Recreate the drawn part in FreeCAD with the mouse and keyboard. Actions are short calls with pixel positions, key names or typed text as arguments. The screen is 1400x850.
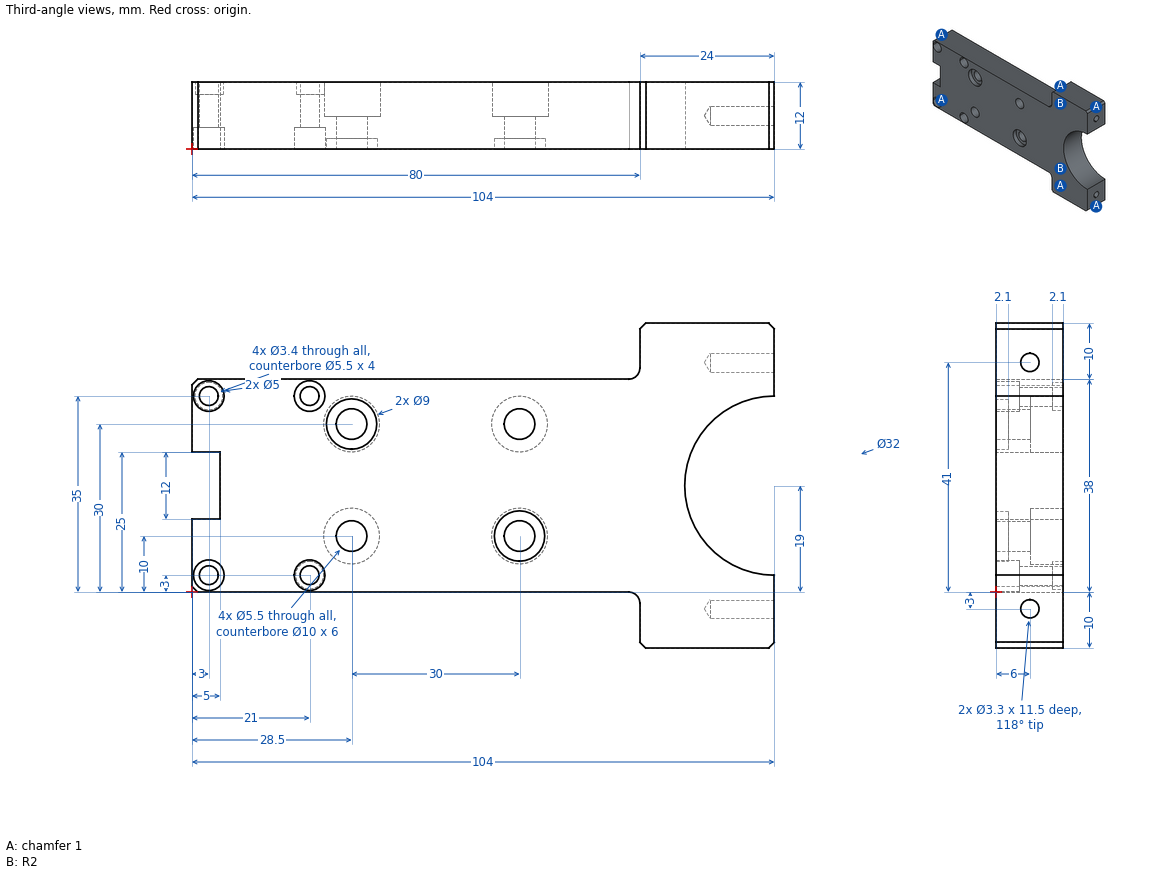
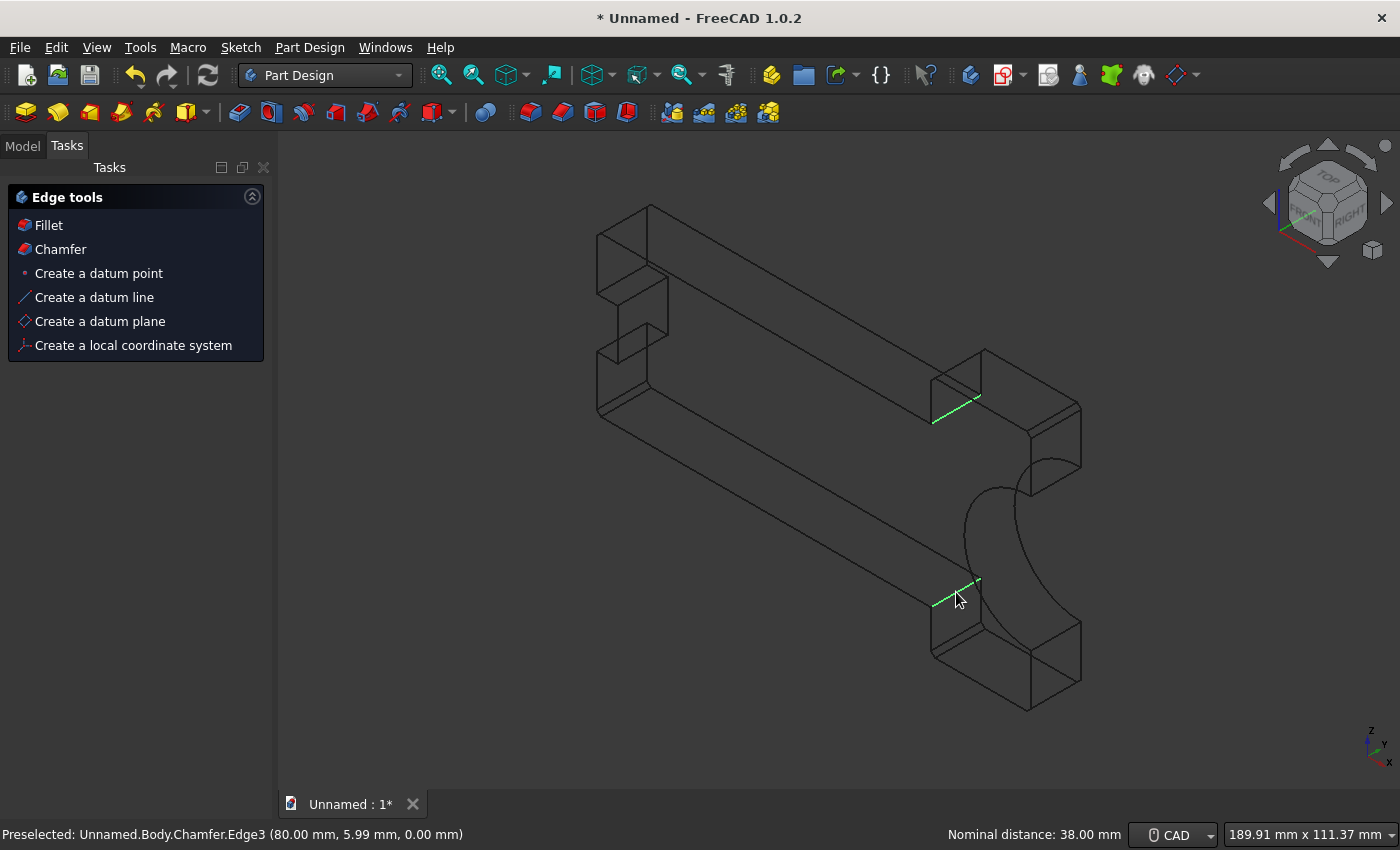
key(v)
key(1)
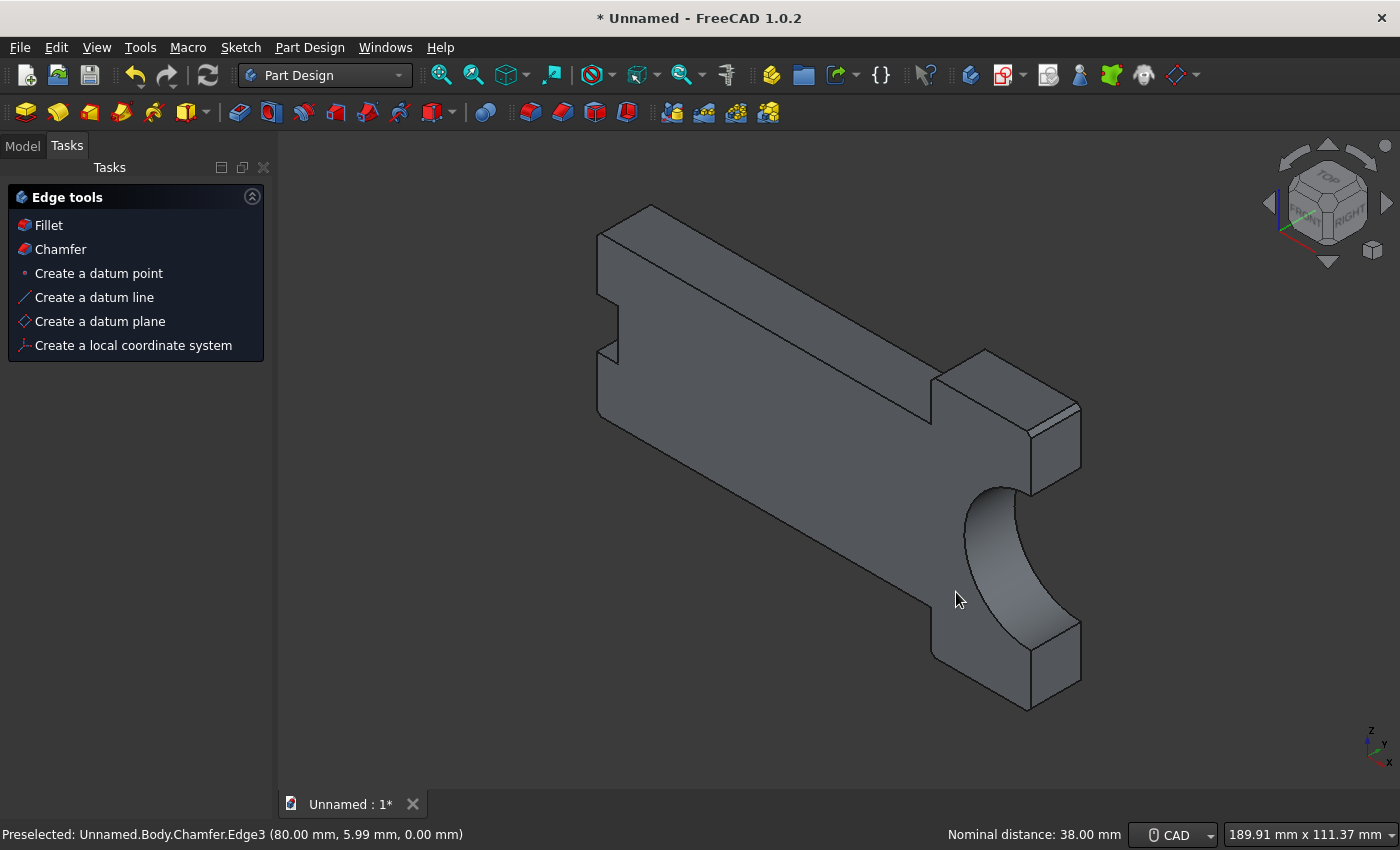
click(532, 112)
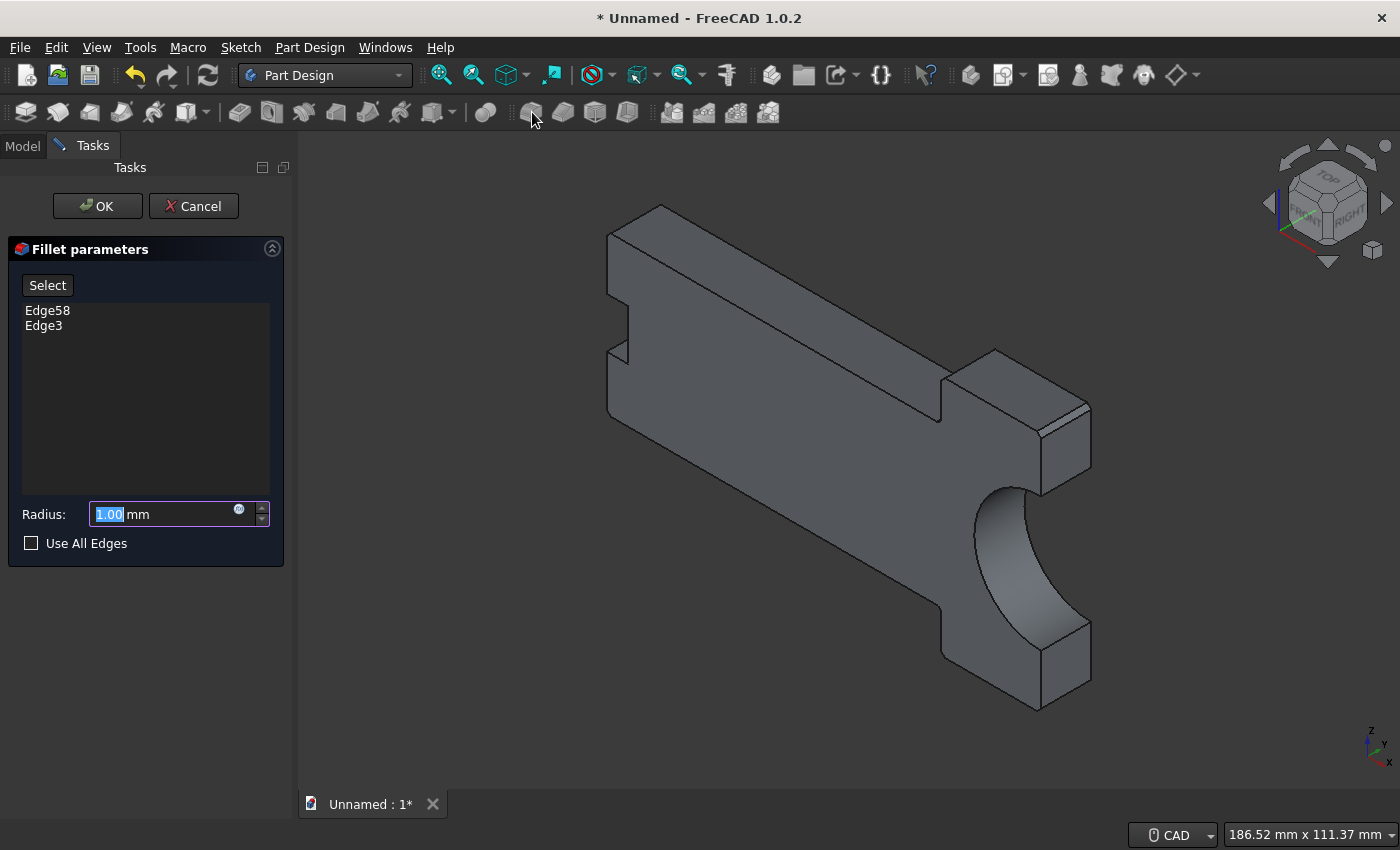
text(2)
key(Tab)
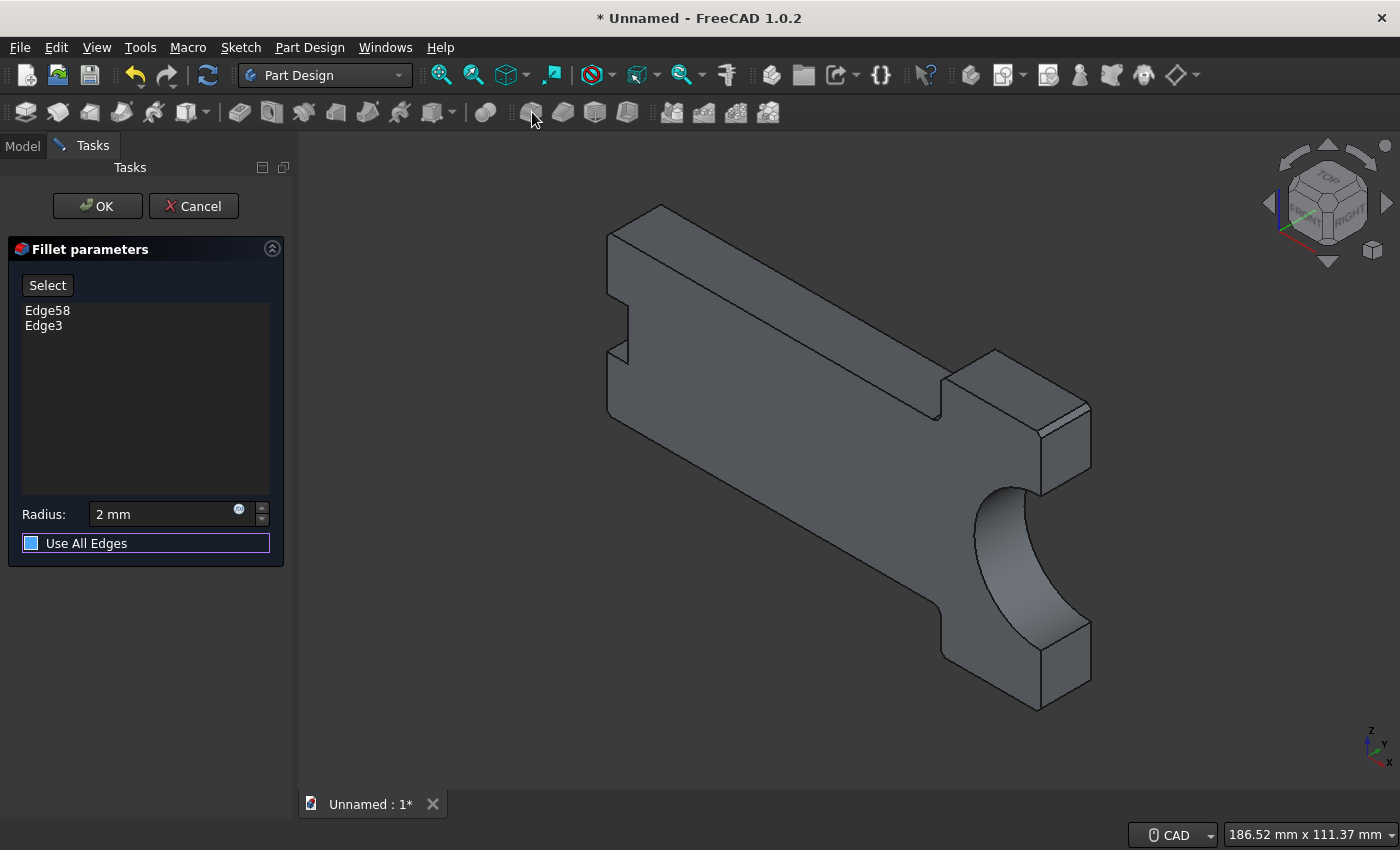
click(98, 206)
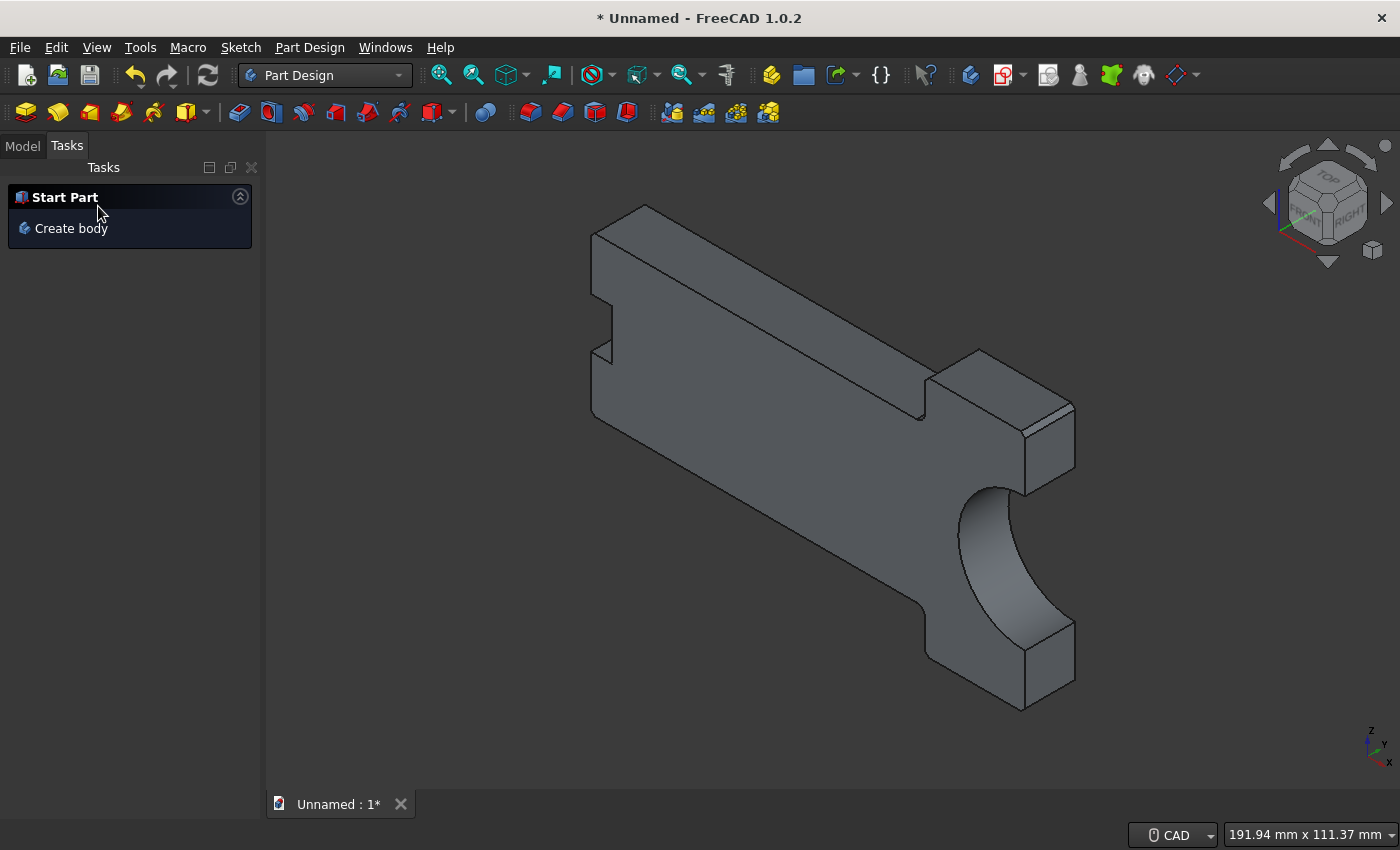
click(1004, 76)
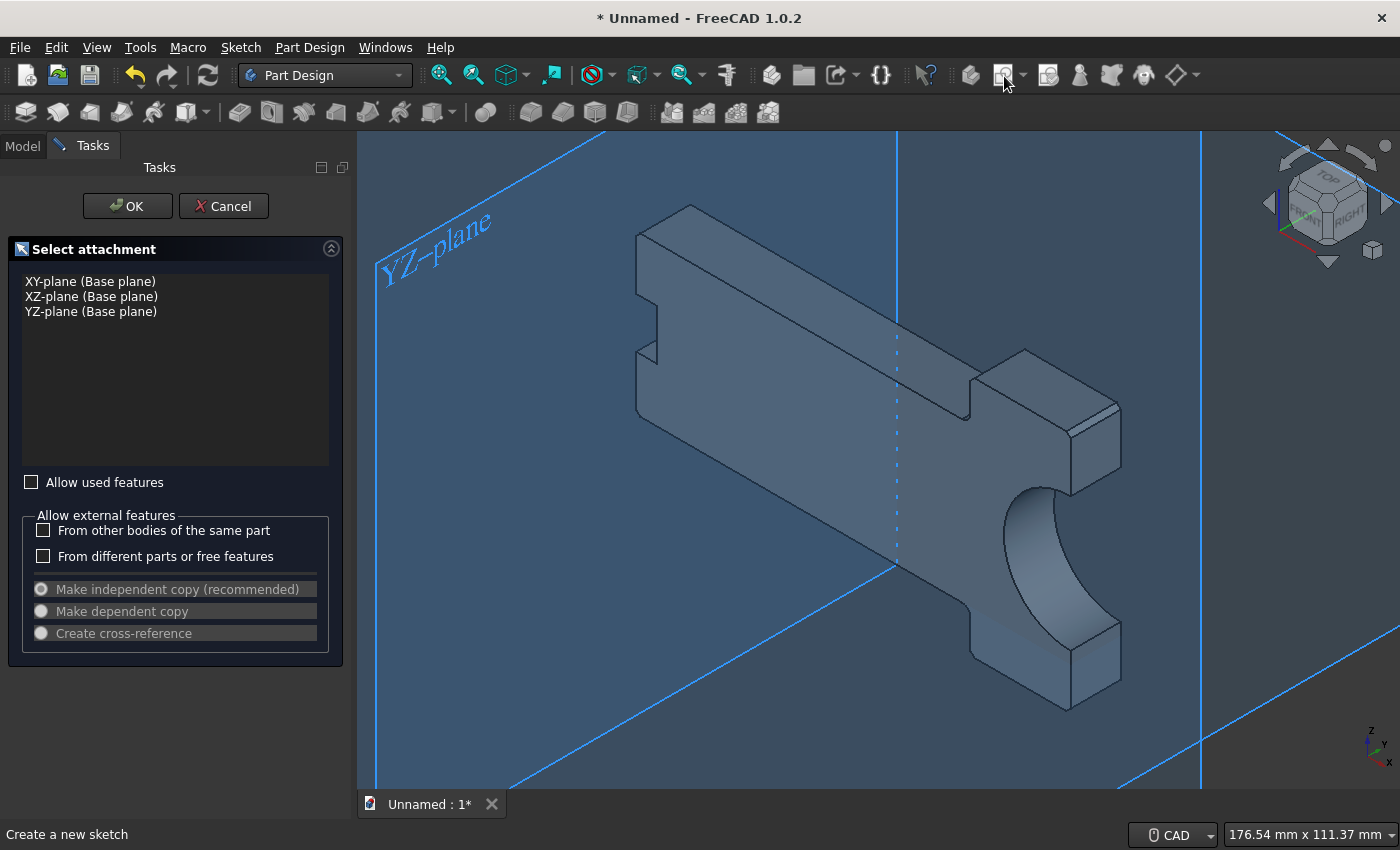
click(82, 296)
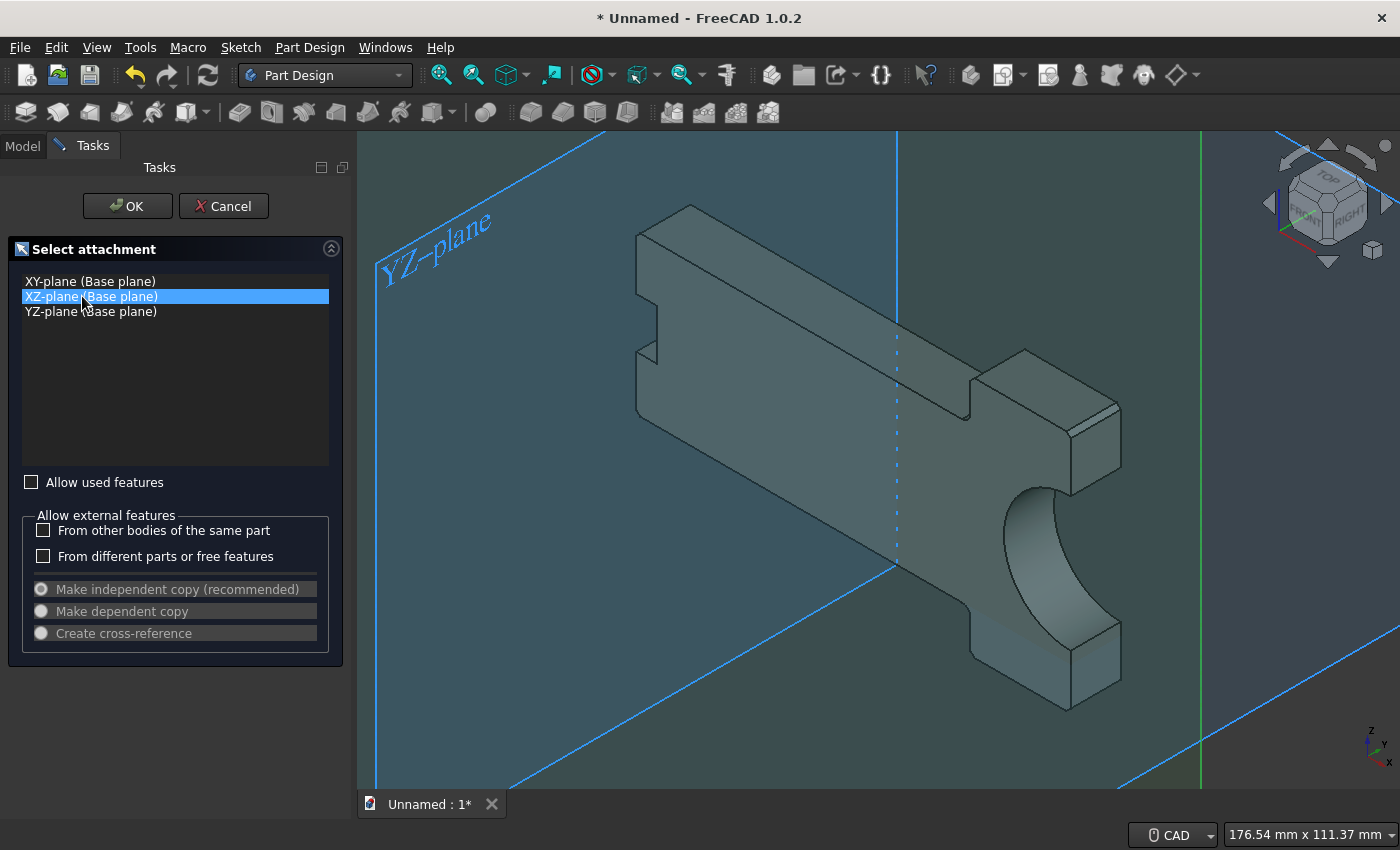
click(128, 206)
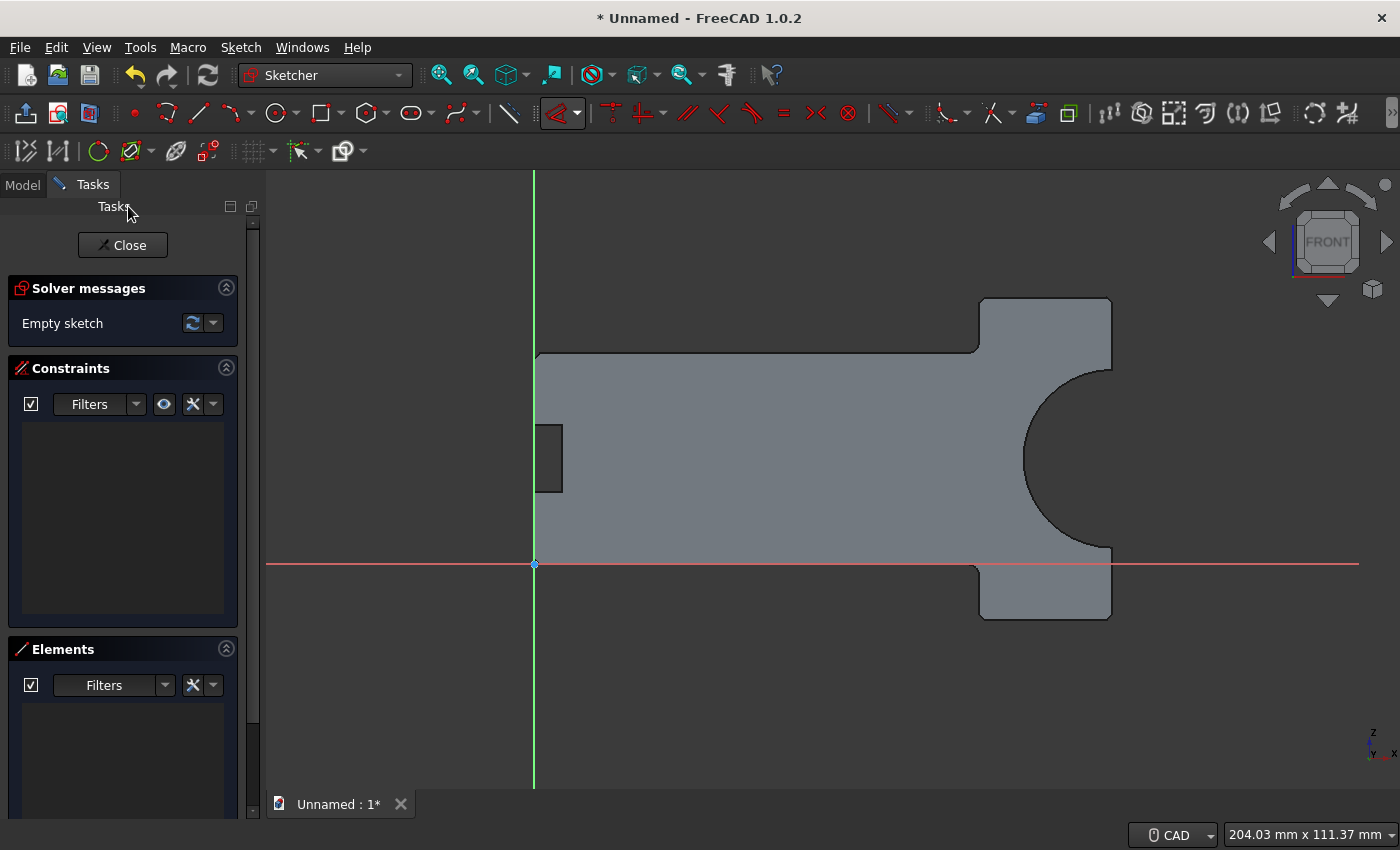
scroll(394, 442, up, 3)